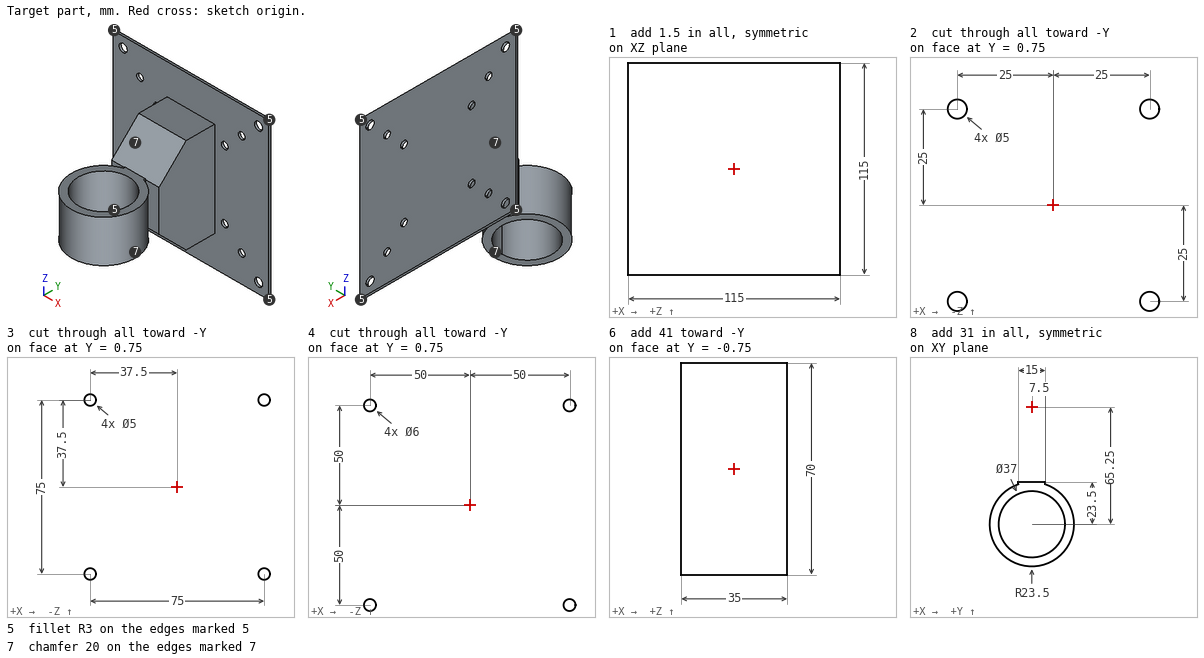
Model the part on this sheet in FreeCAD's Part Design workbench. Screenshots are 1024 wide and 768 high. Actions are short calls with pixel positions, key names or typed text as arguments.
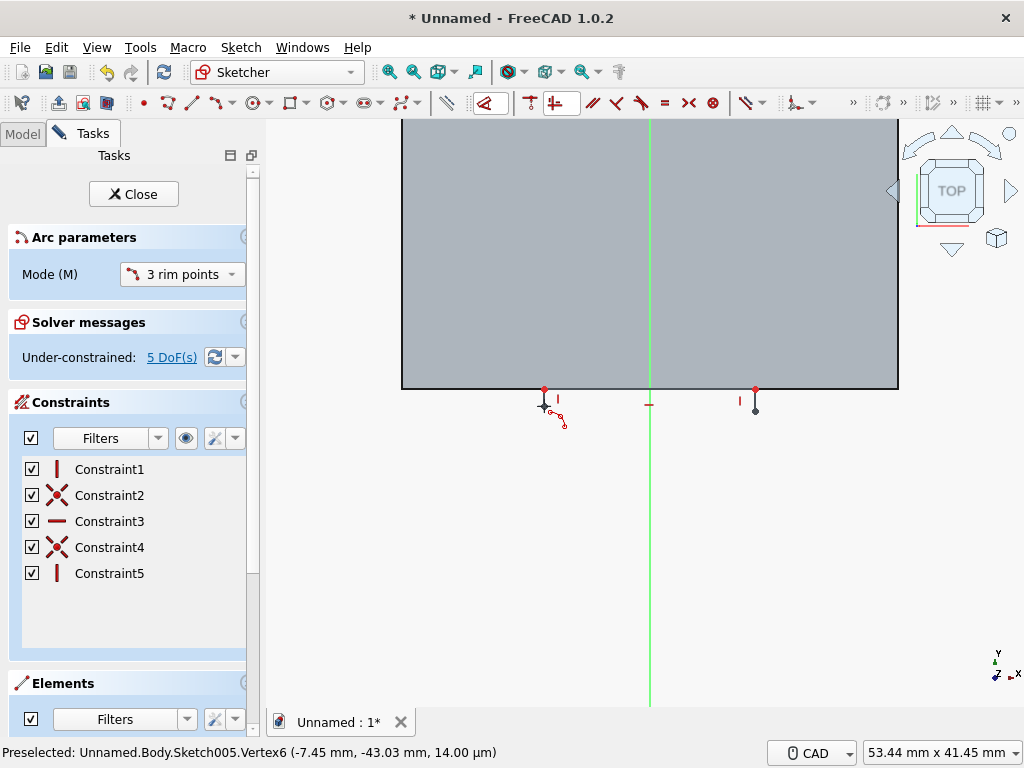
scroll(543, 406, up, 3)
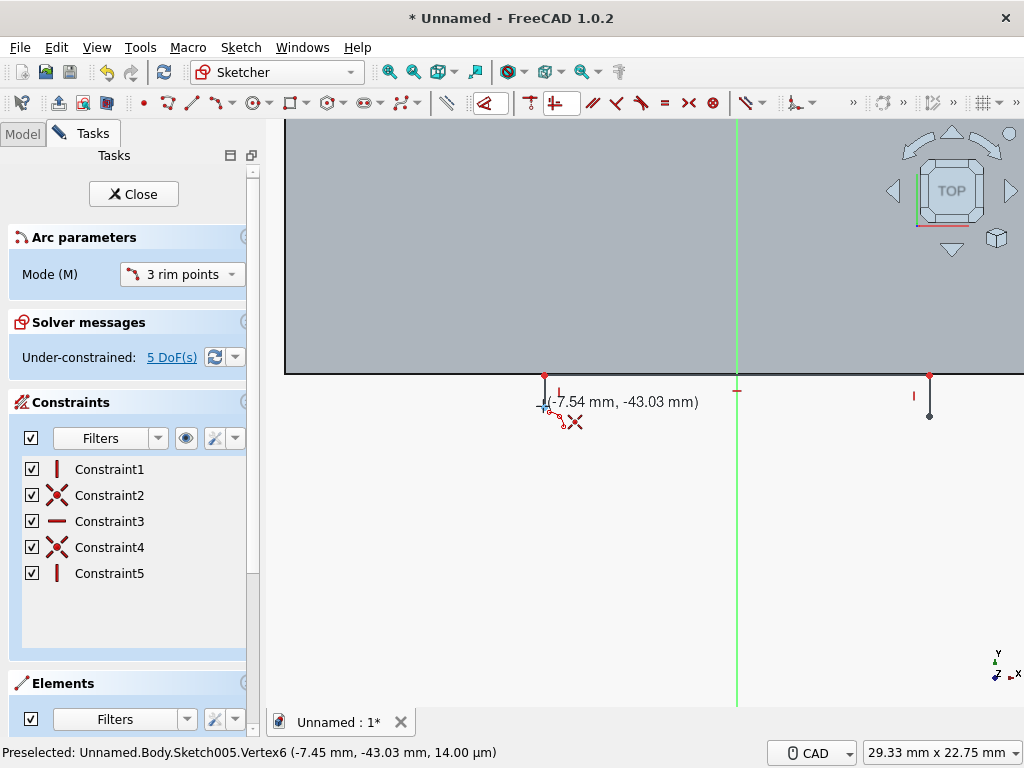
click(545, 407)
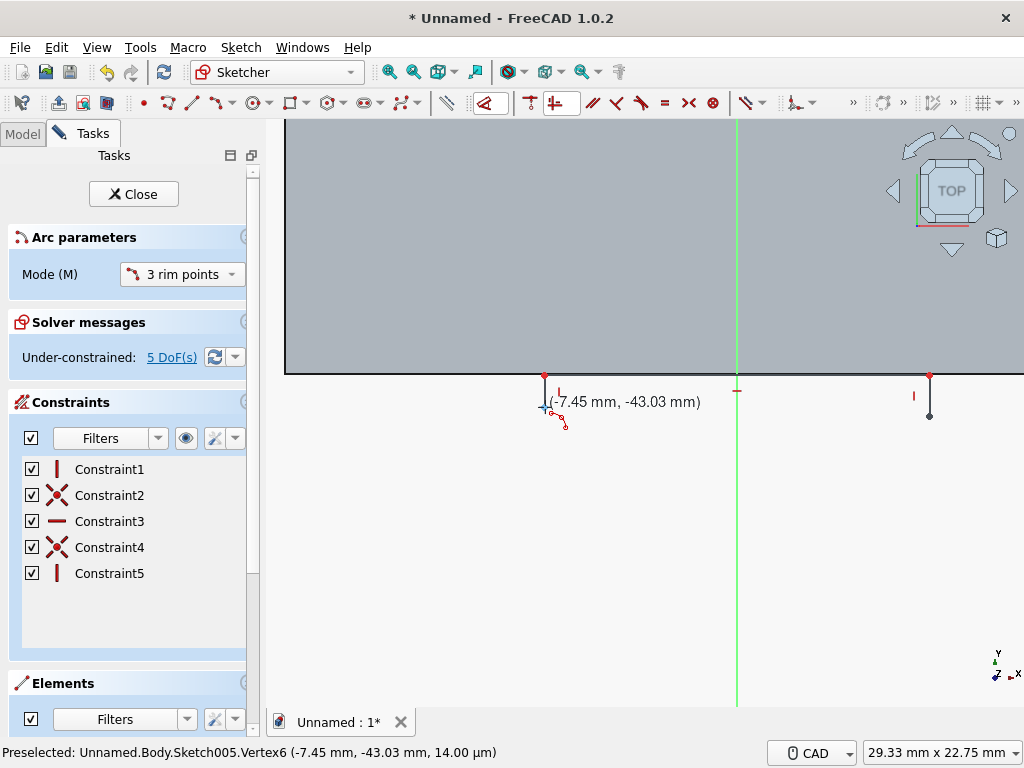
scroll(545, 407, down, 9)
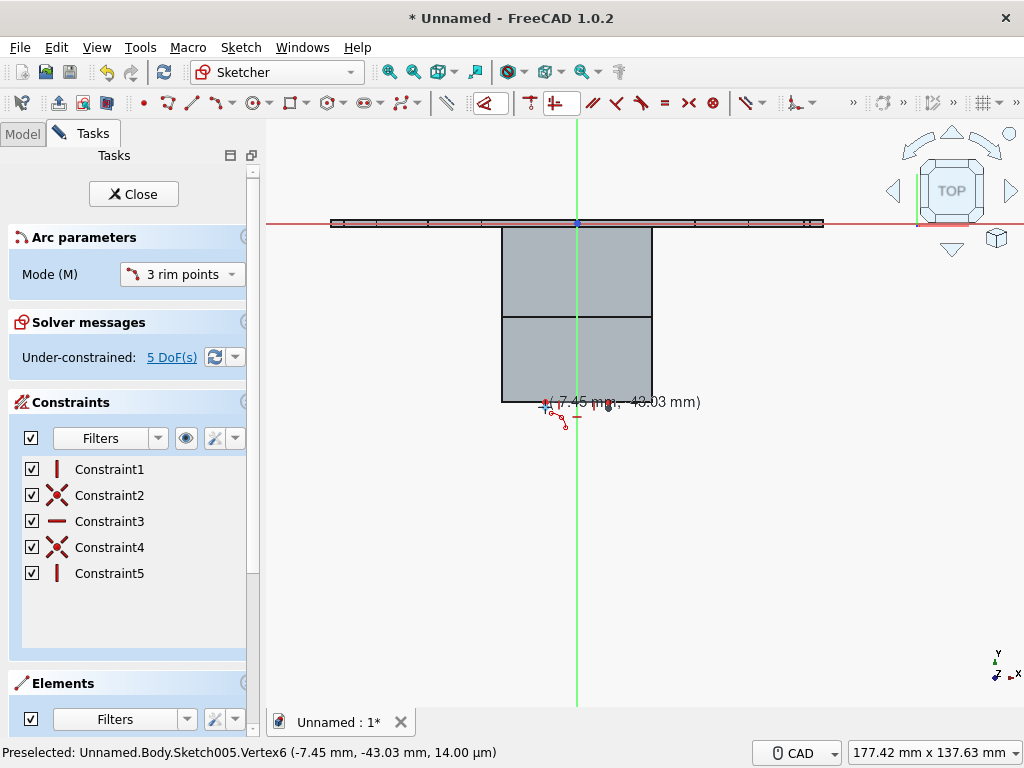
scroll(609, 407, up, 9)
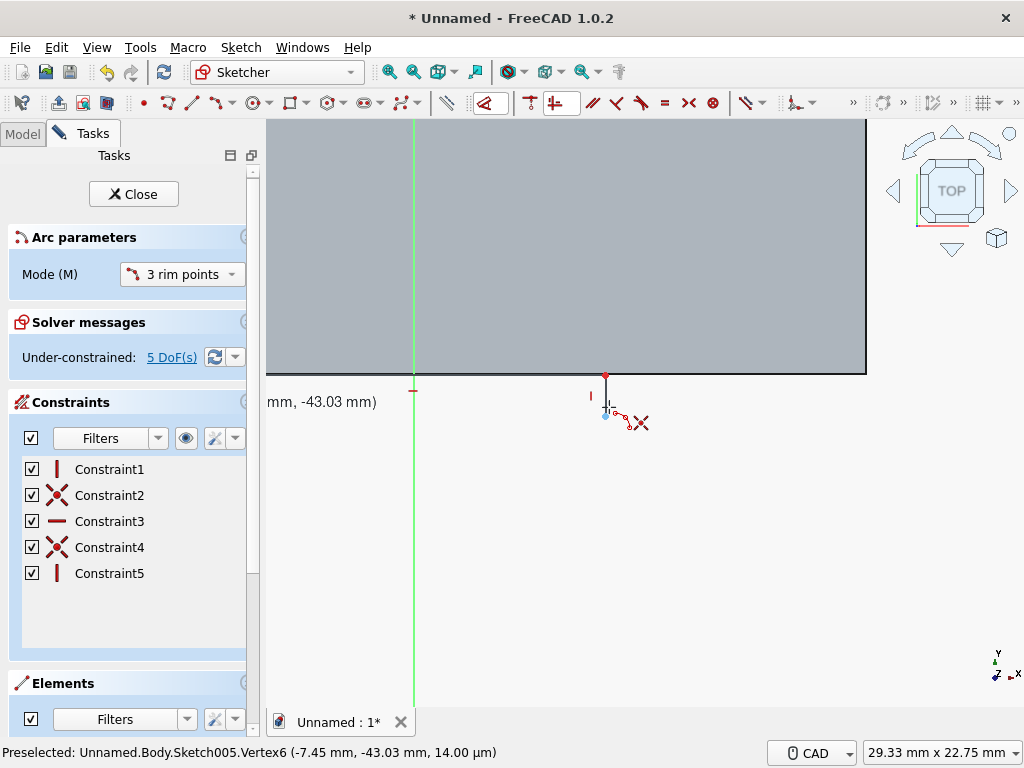
click(606, 416)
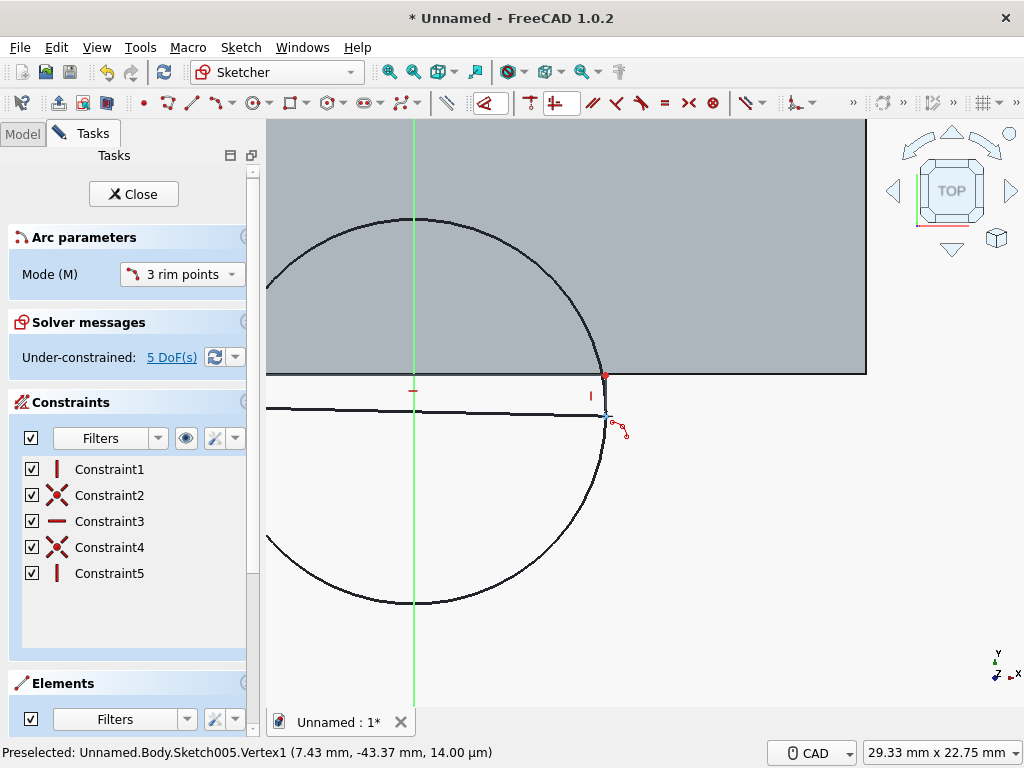
scroll(609, 407, down, 9)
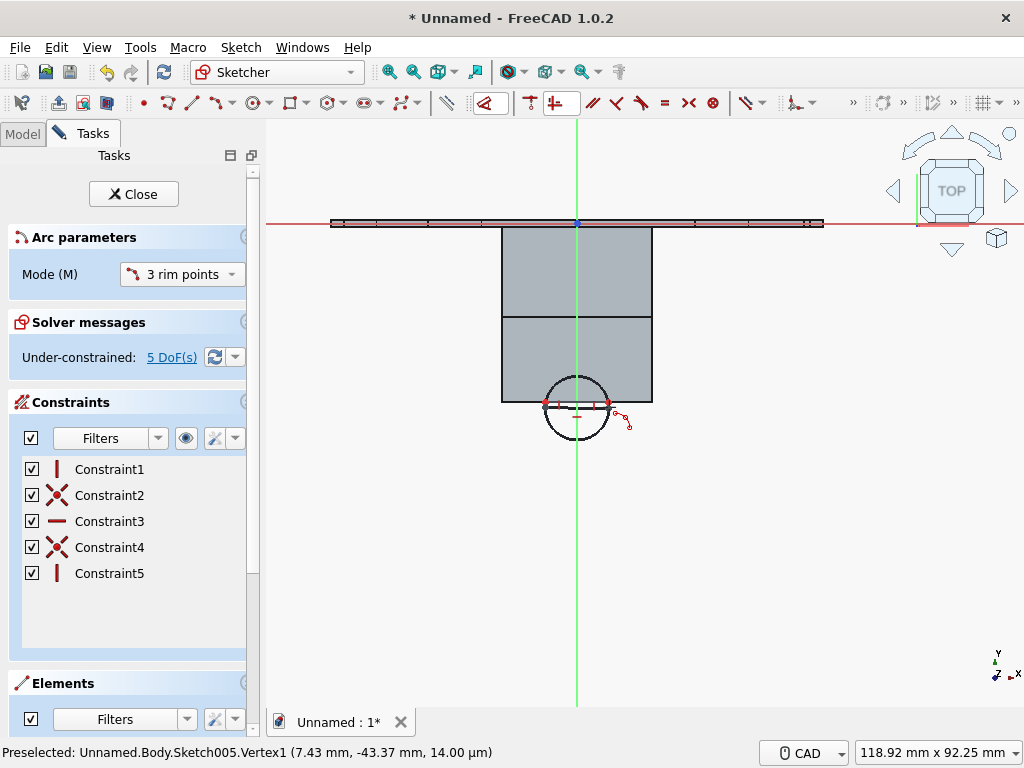
click(524, 587)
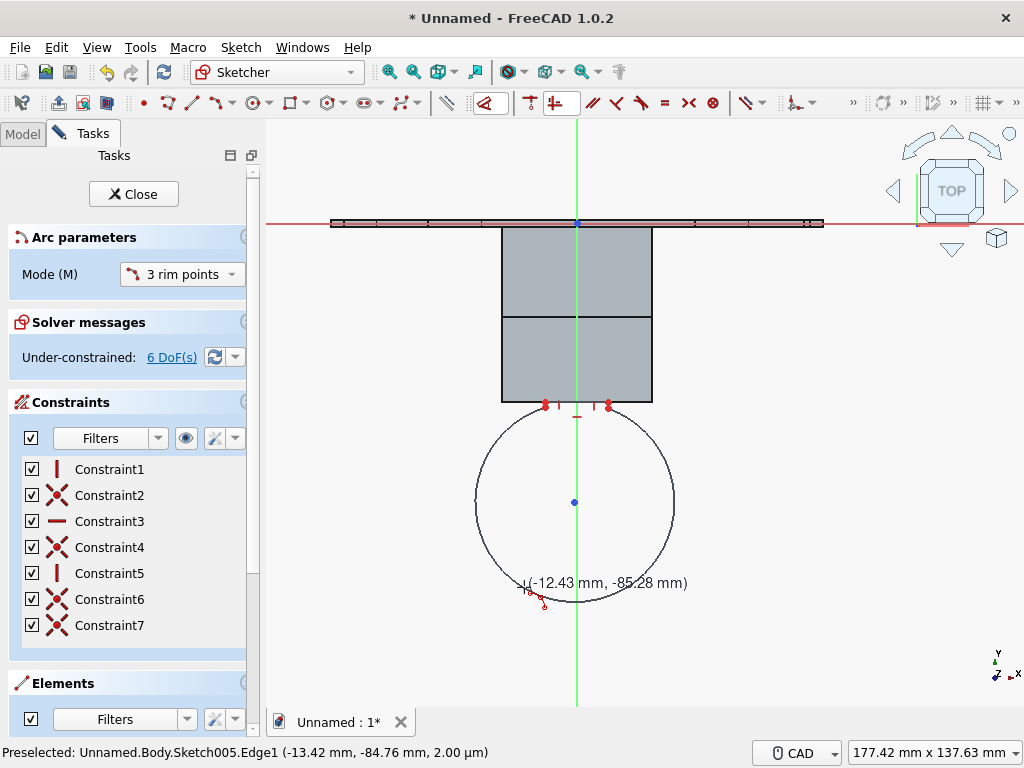
click(254, 104)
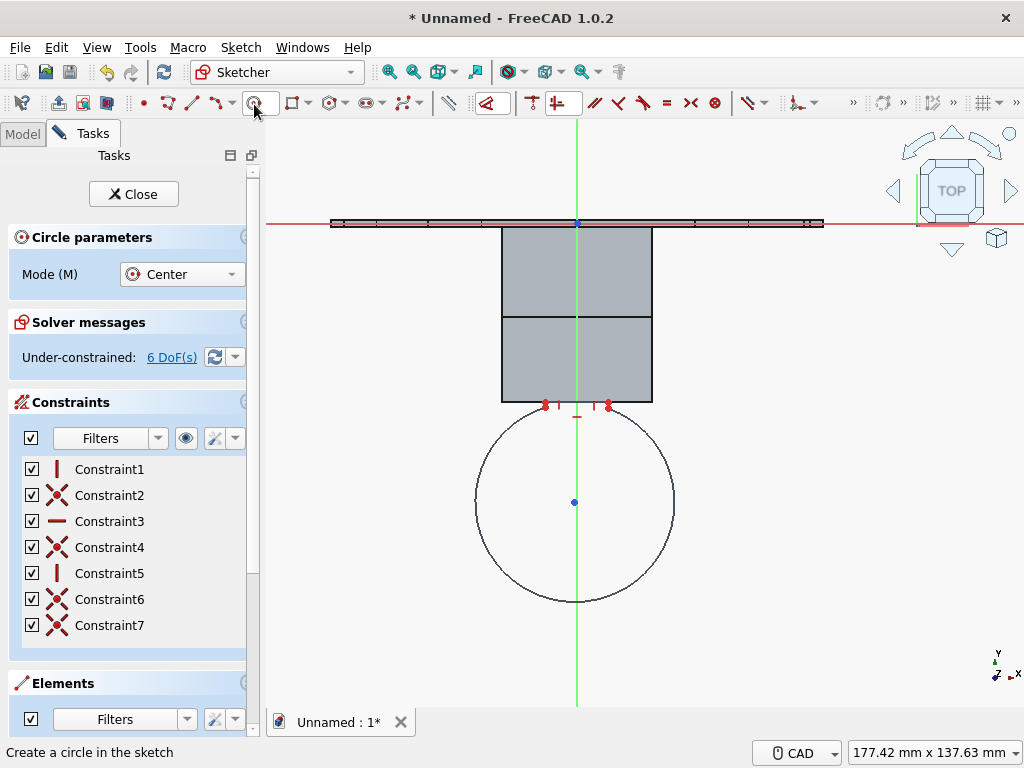
click(577, 502)
click(633, 447)
key(Escape)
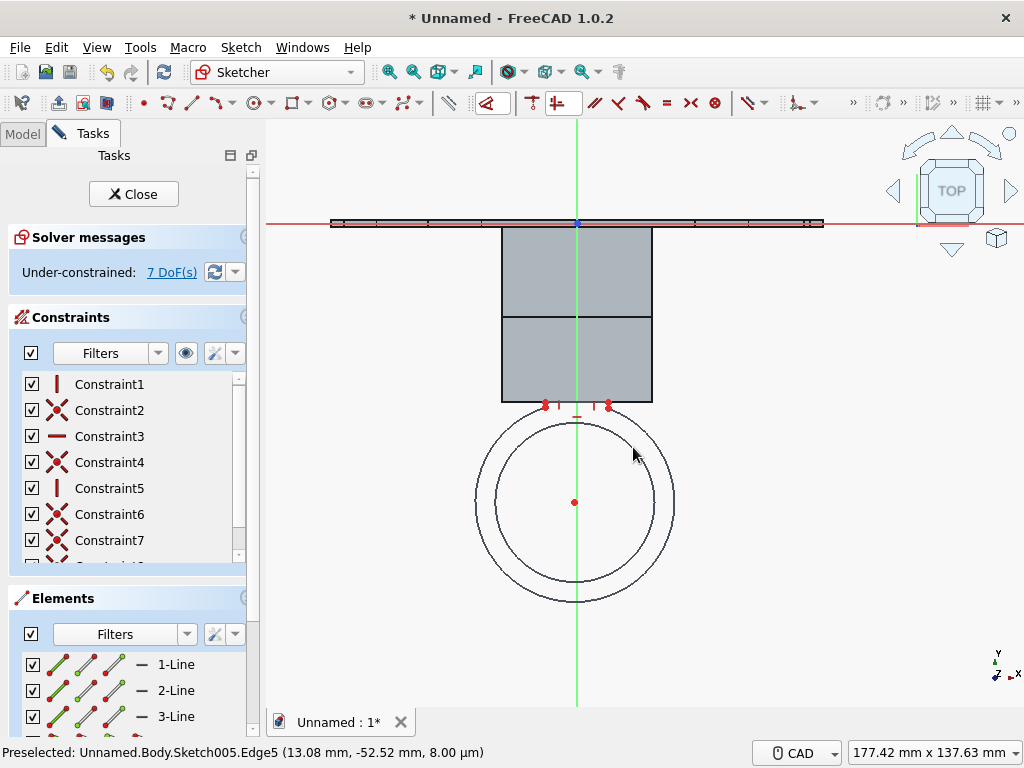
click(575, 502)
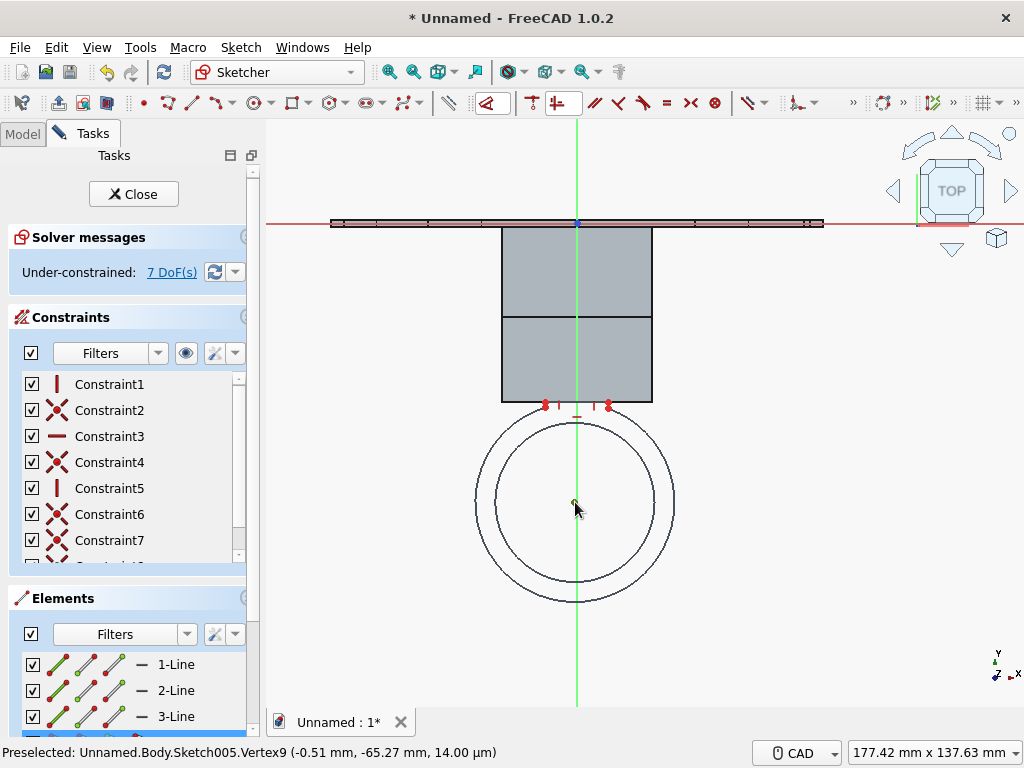
click(577, 641)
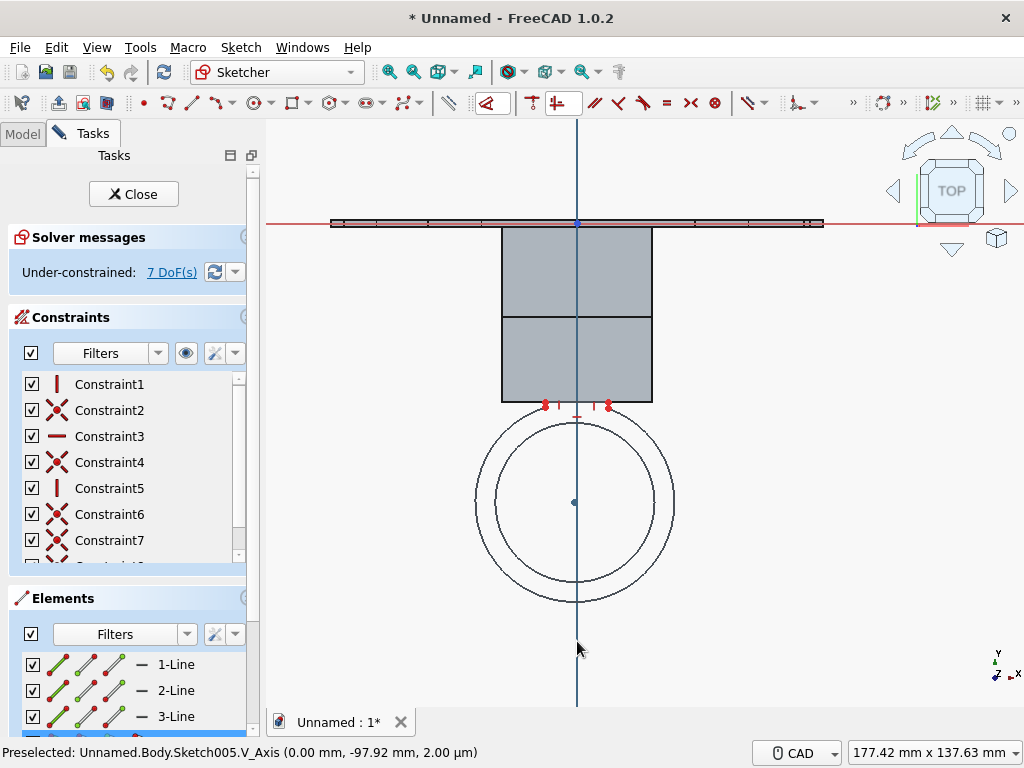
key(c)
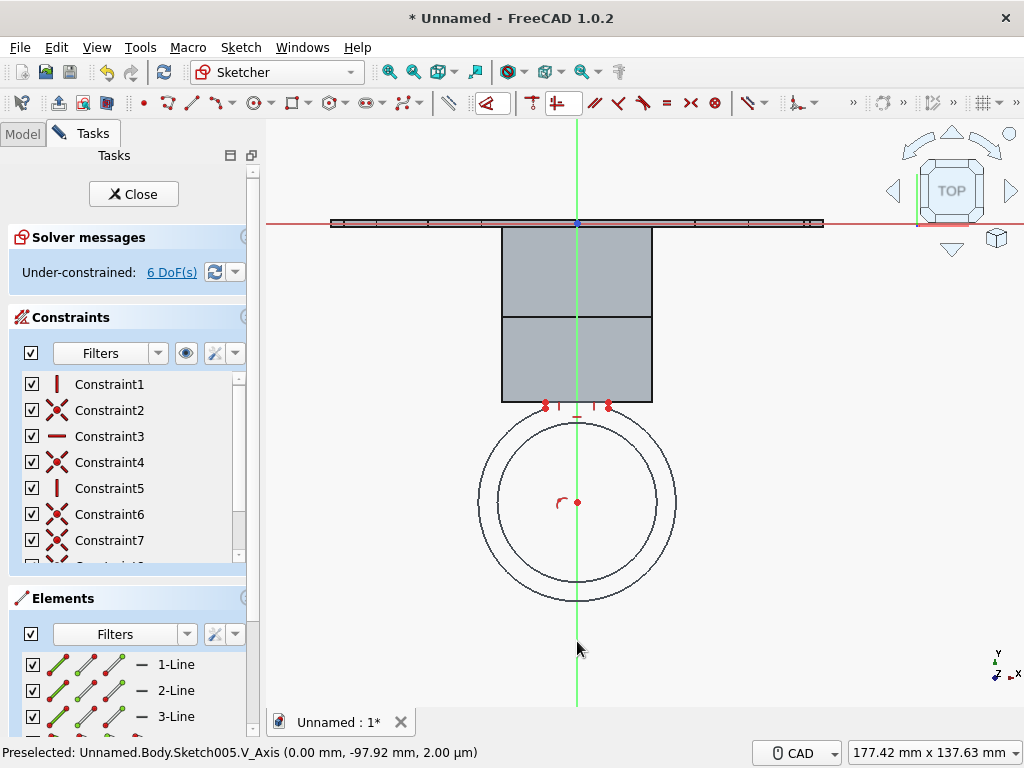
key(d)